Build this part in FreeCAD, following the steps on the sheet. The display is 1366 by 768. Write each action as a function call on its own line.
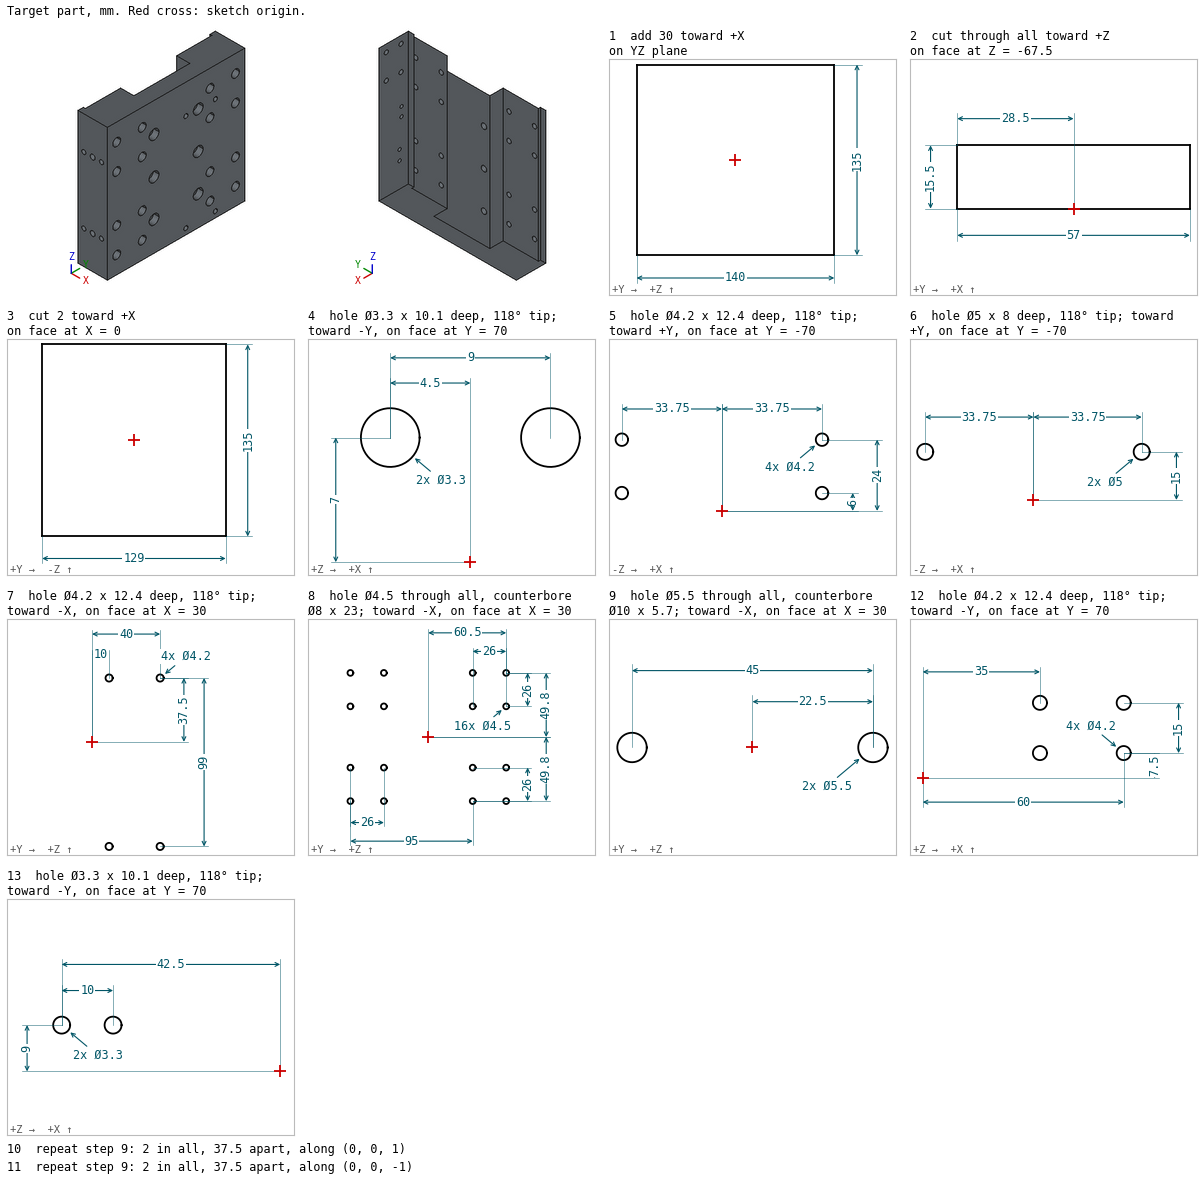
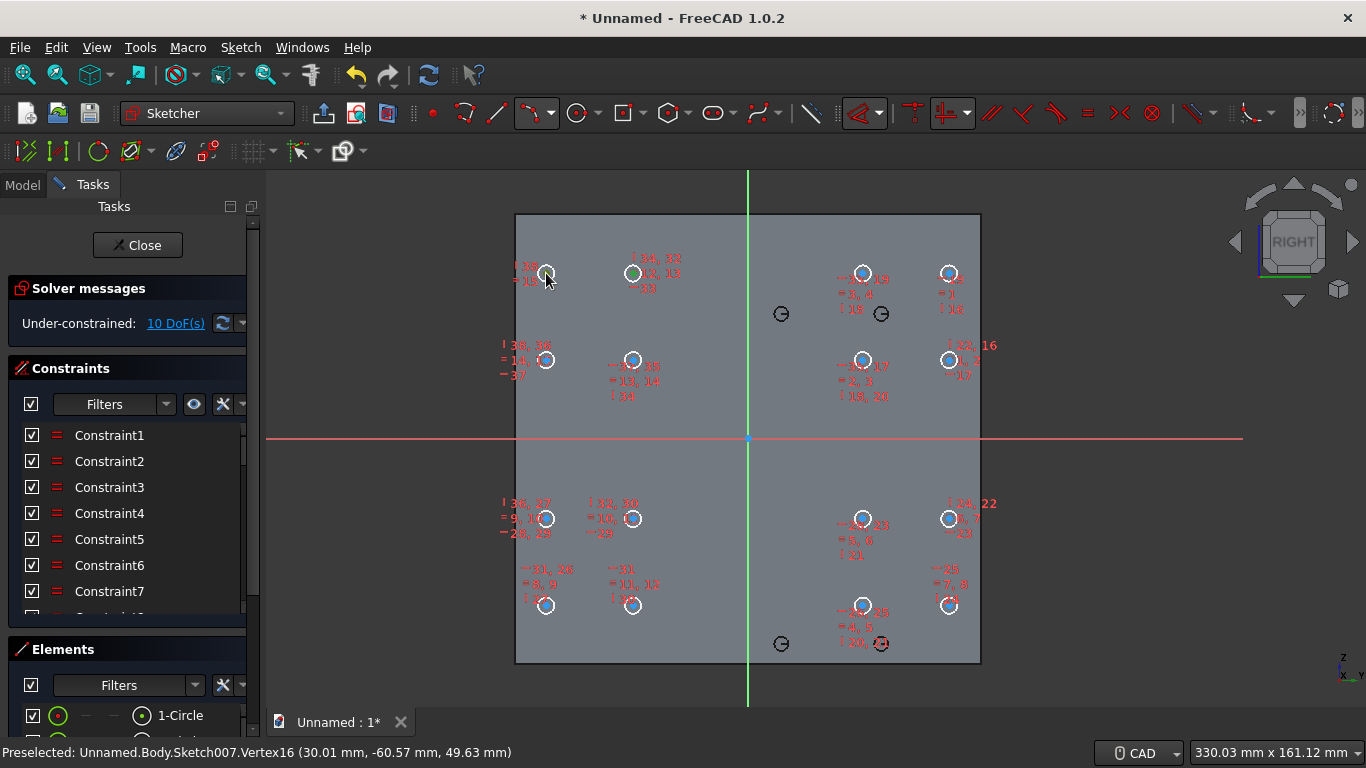
click(970, 114)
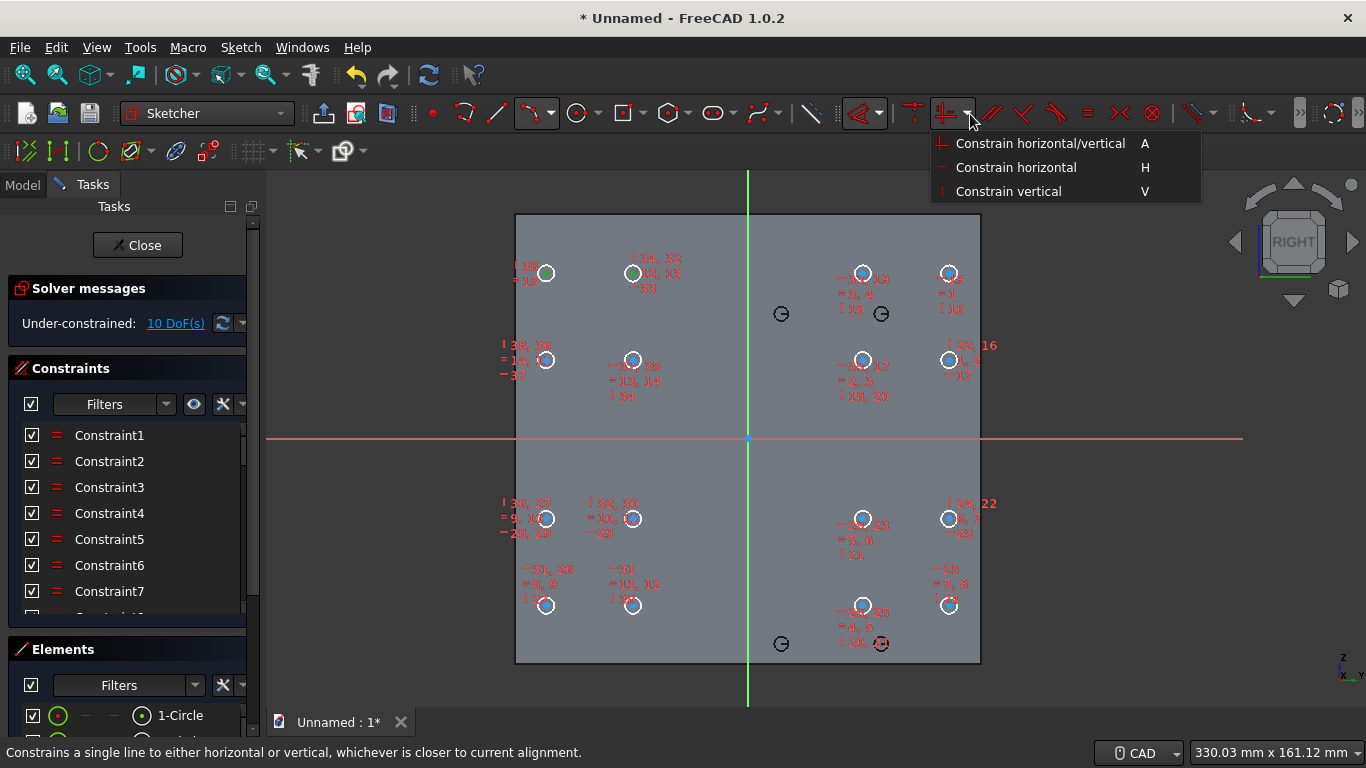
click(1066, 167)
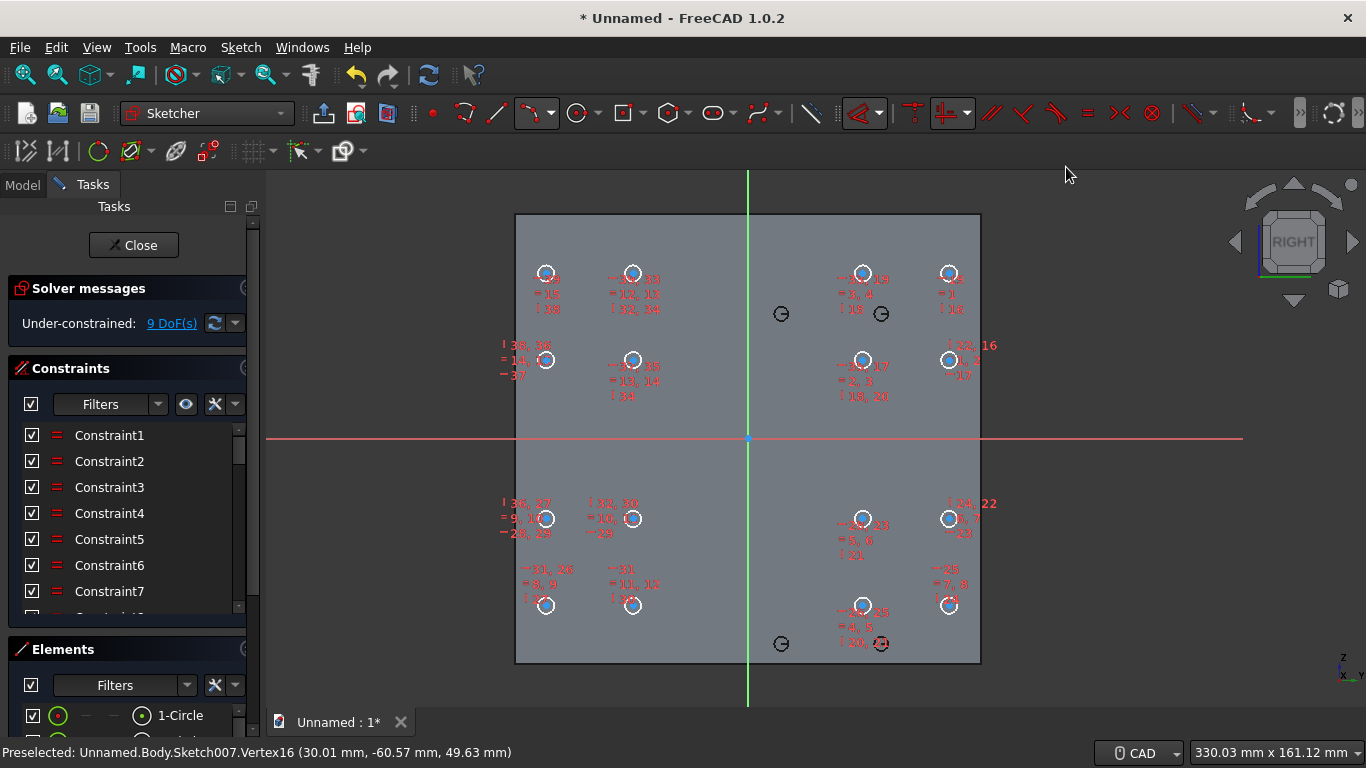
scroll(955, 268, up, 5)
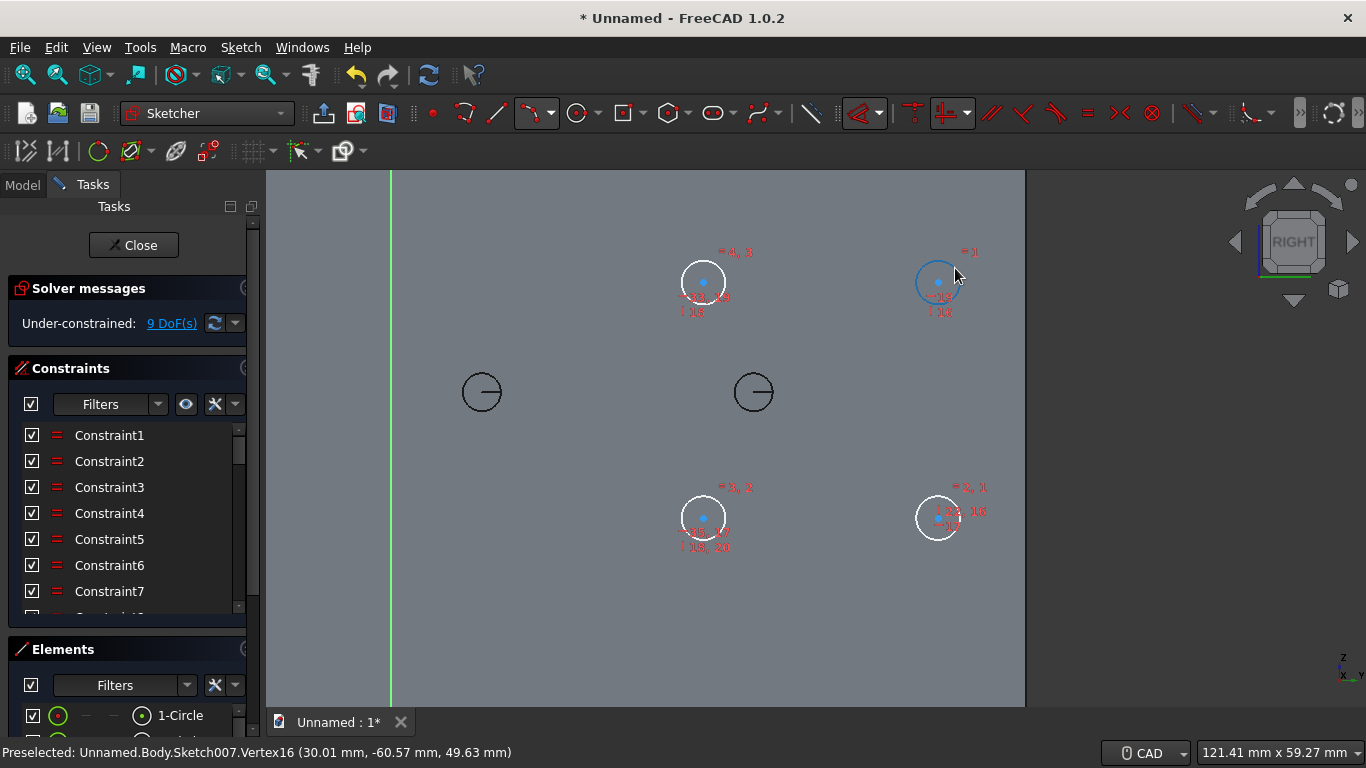
click(953, 267)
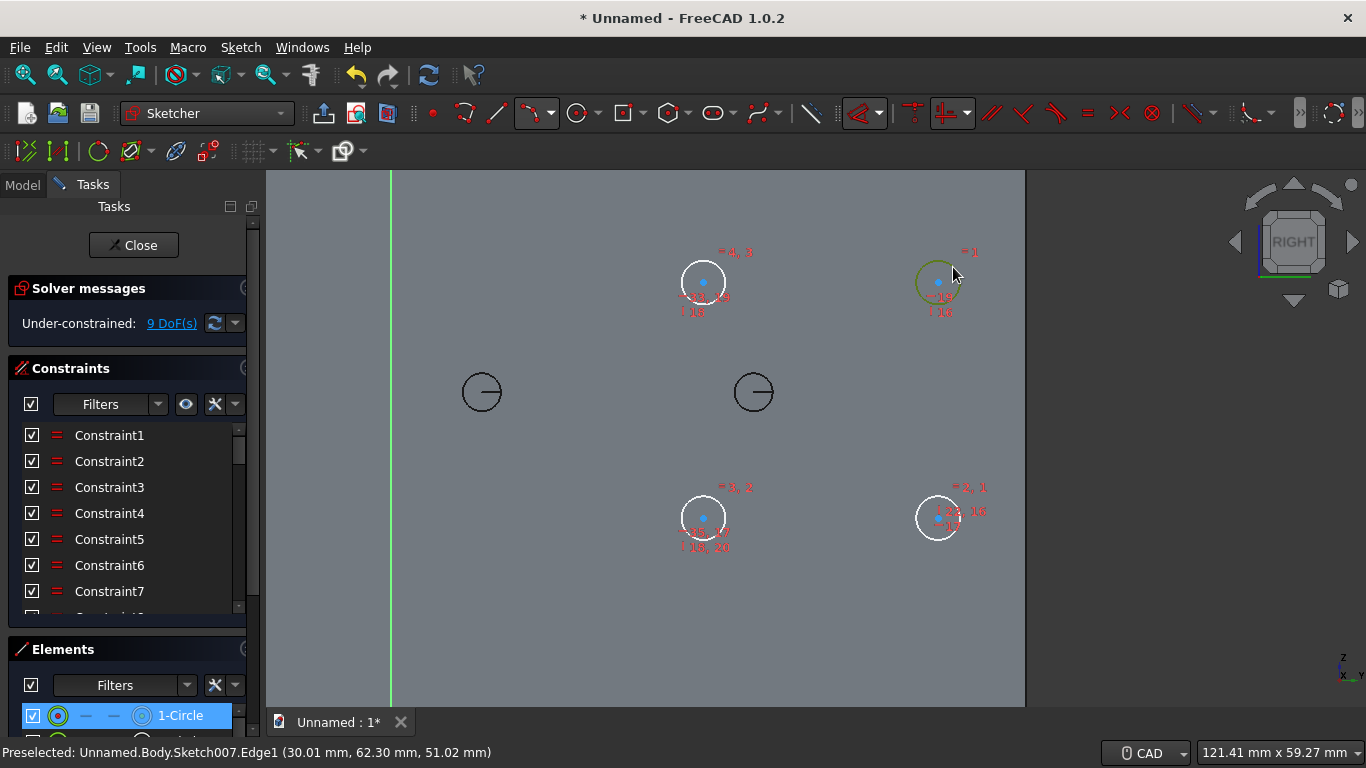
click(882, 114)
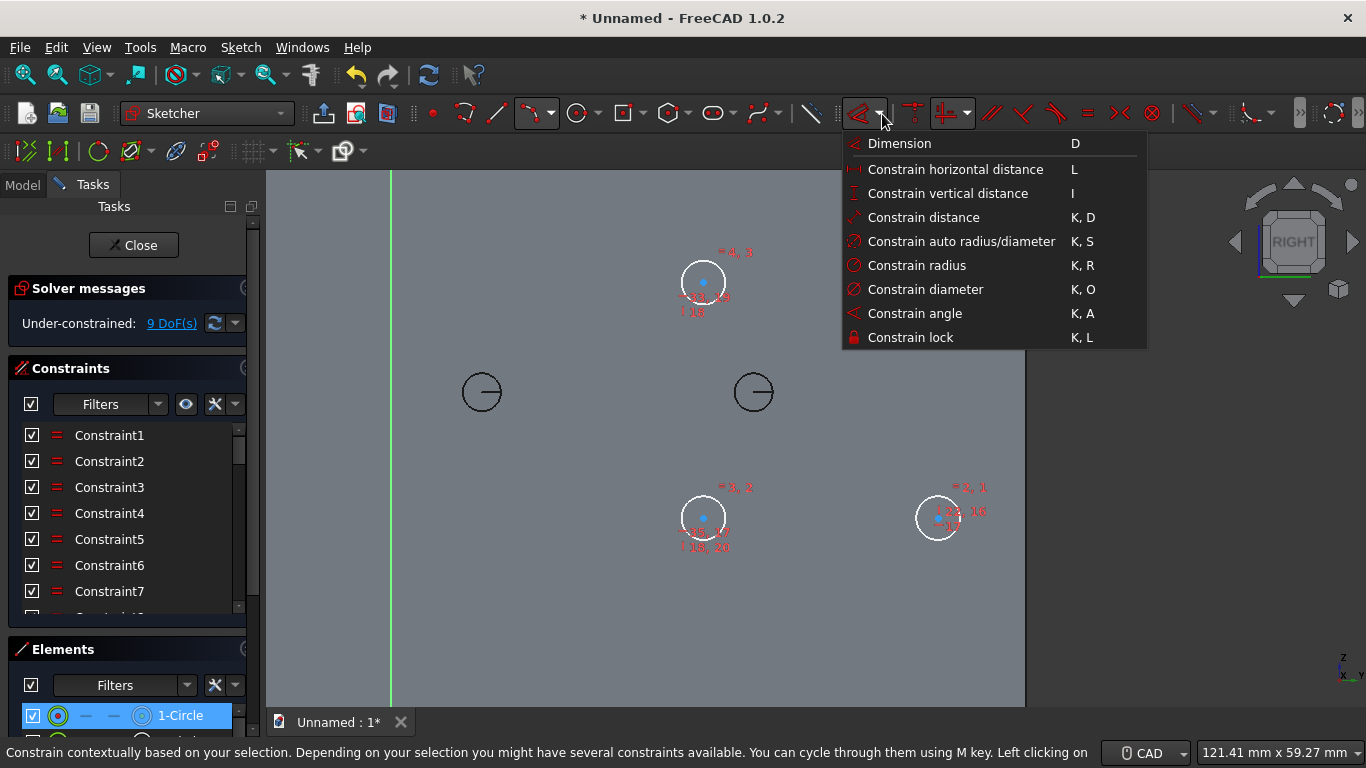
click(995, 289)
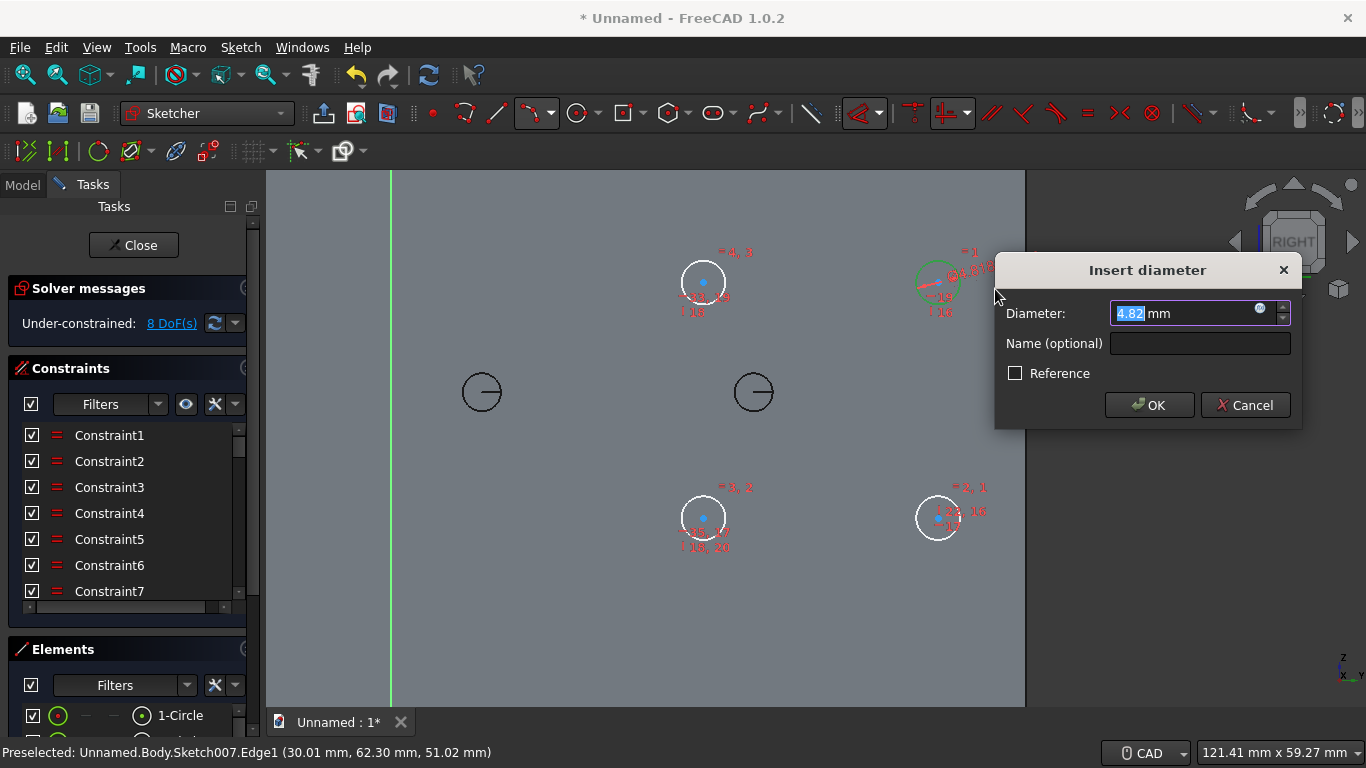
text(4.5)
key(Return)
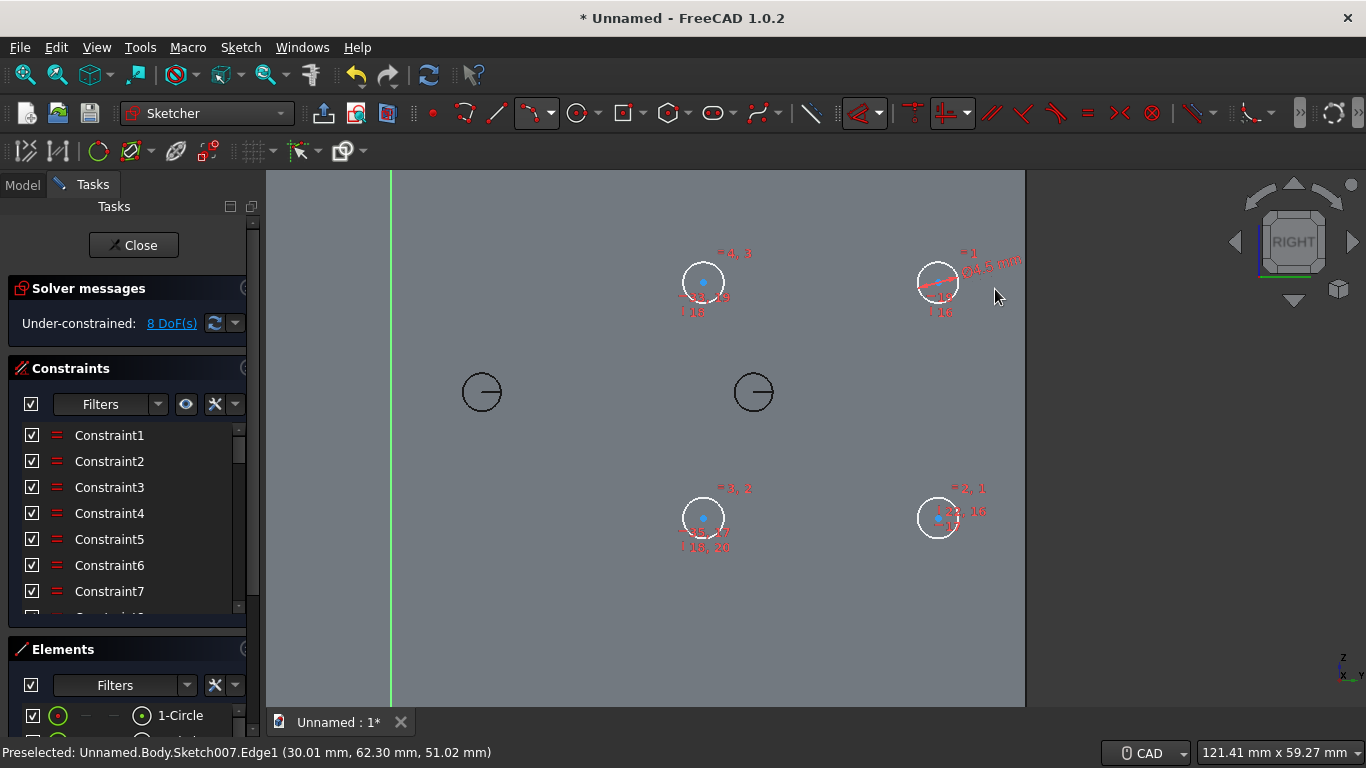
click(938, 283)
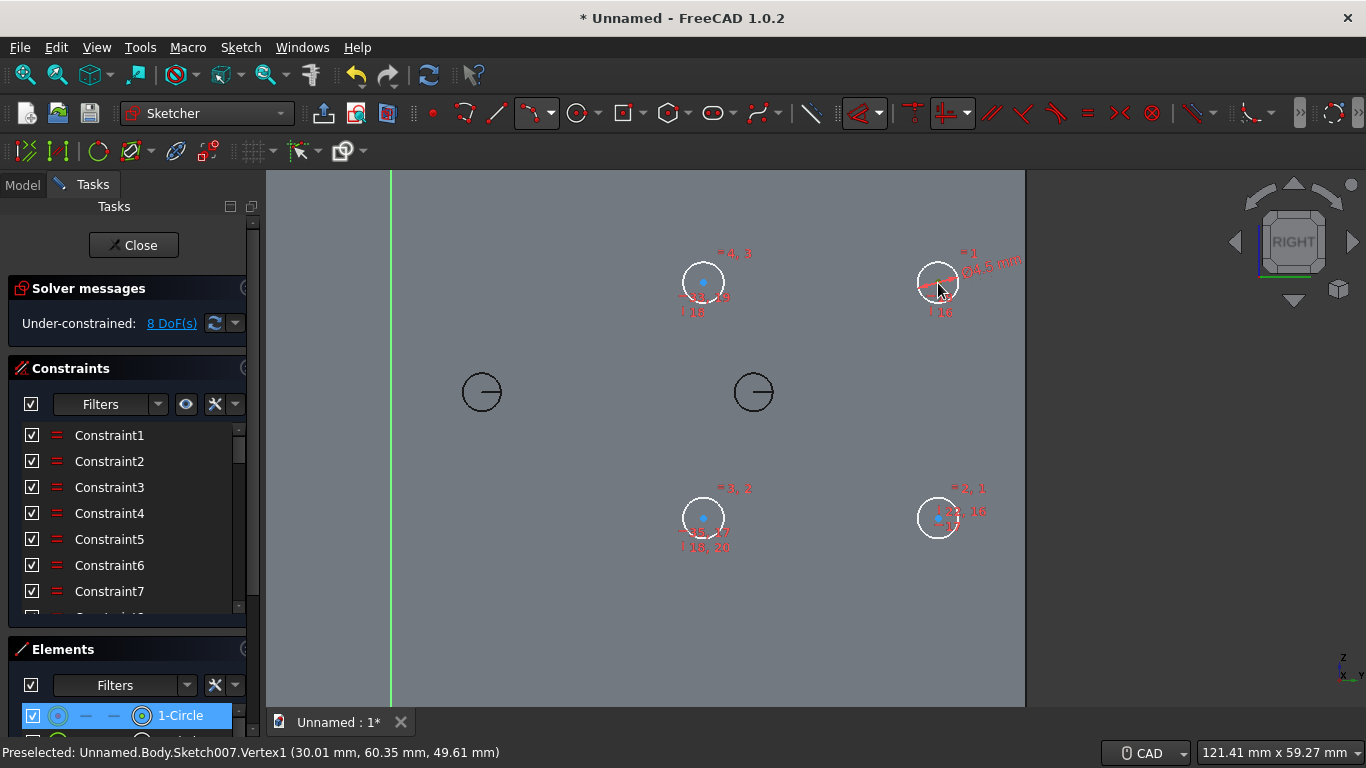
click(938, 518)